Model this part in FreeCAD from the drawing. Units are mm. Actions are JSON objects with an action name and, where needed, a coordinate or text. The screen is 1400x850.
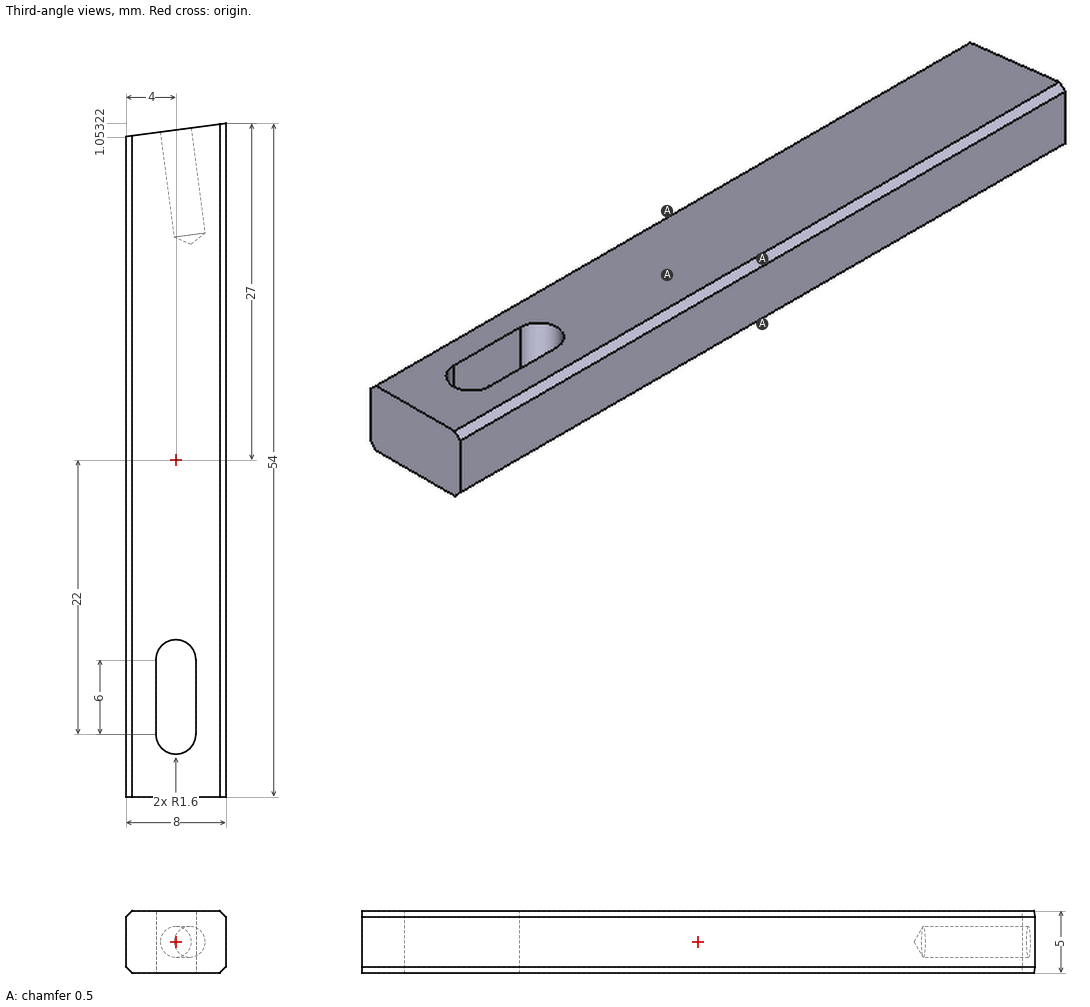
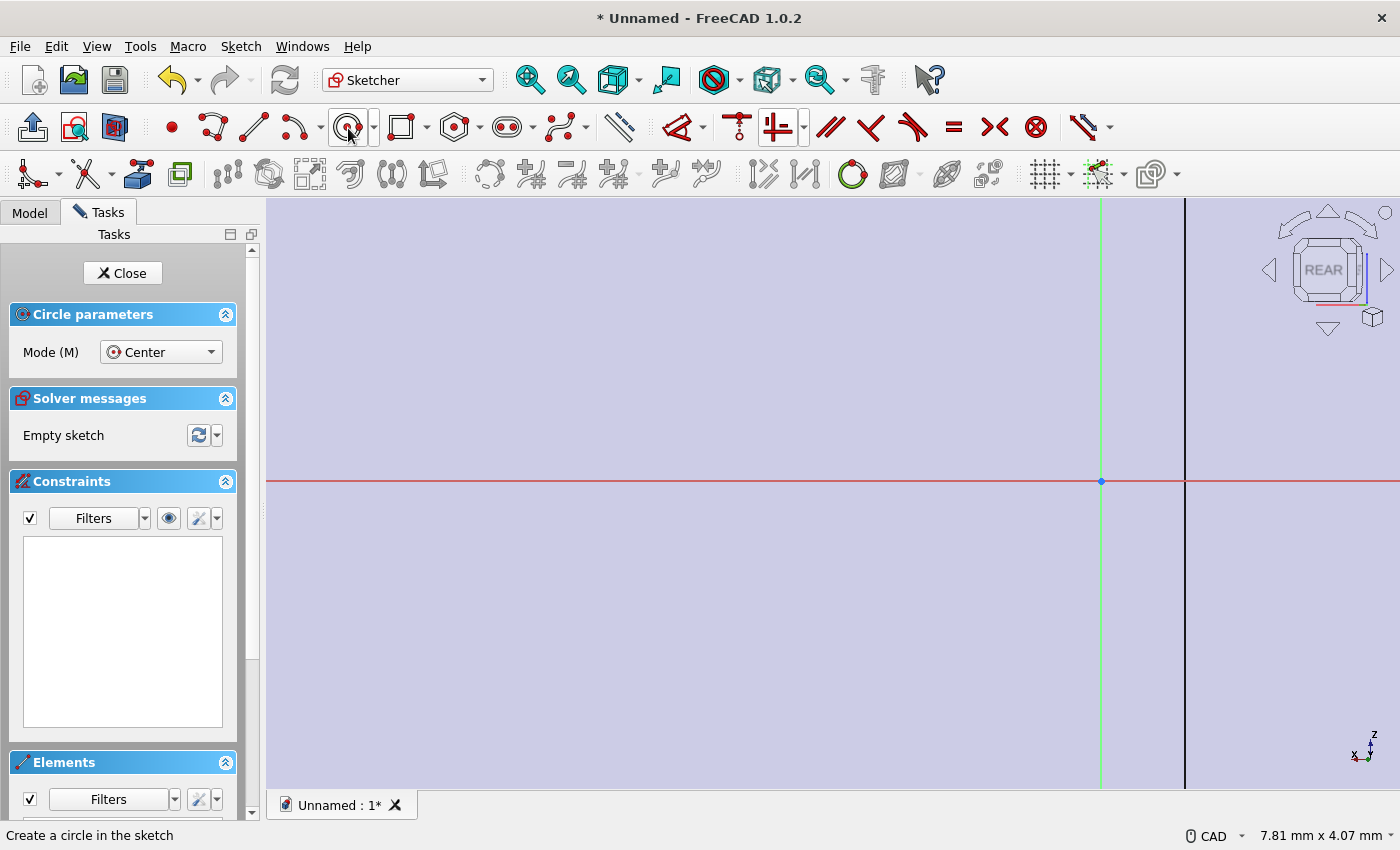
{"action": "left_click", "coordinate": [600, 481]}
{"action": "left_click", "coordinate": [728, 353]}
{"action": "key", "text": "Escape"}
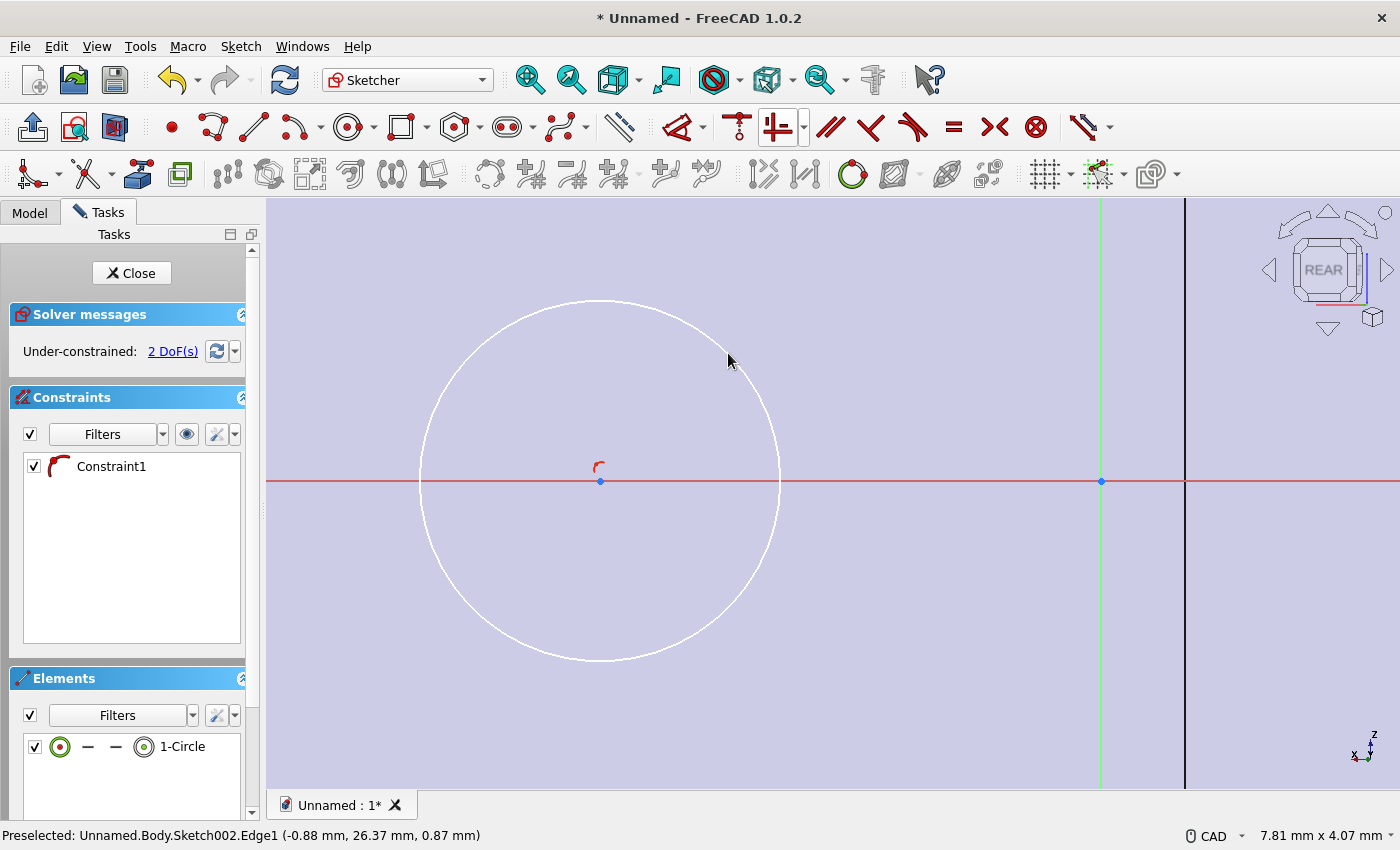
{"action": "left_click", "coordinate": [727, 353]}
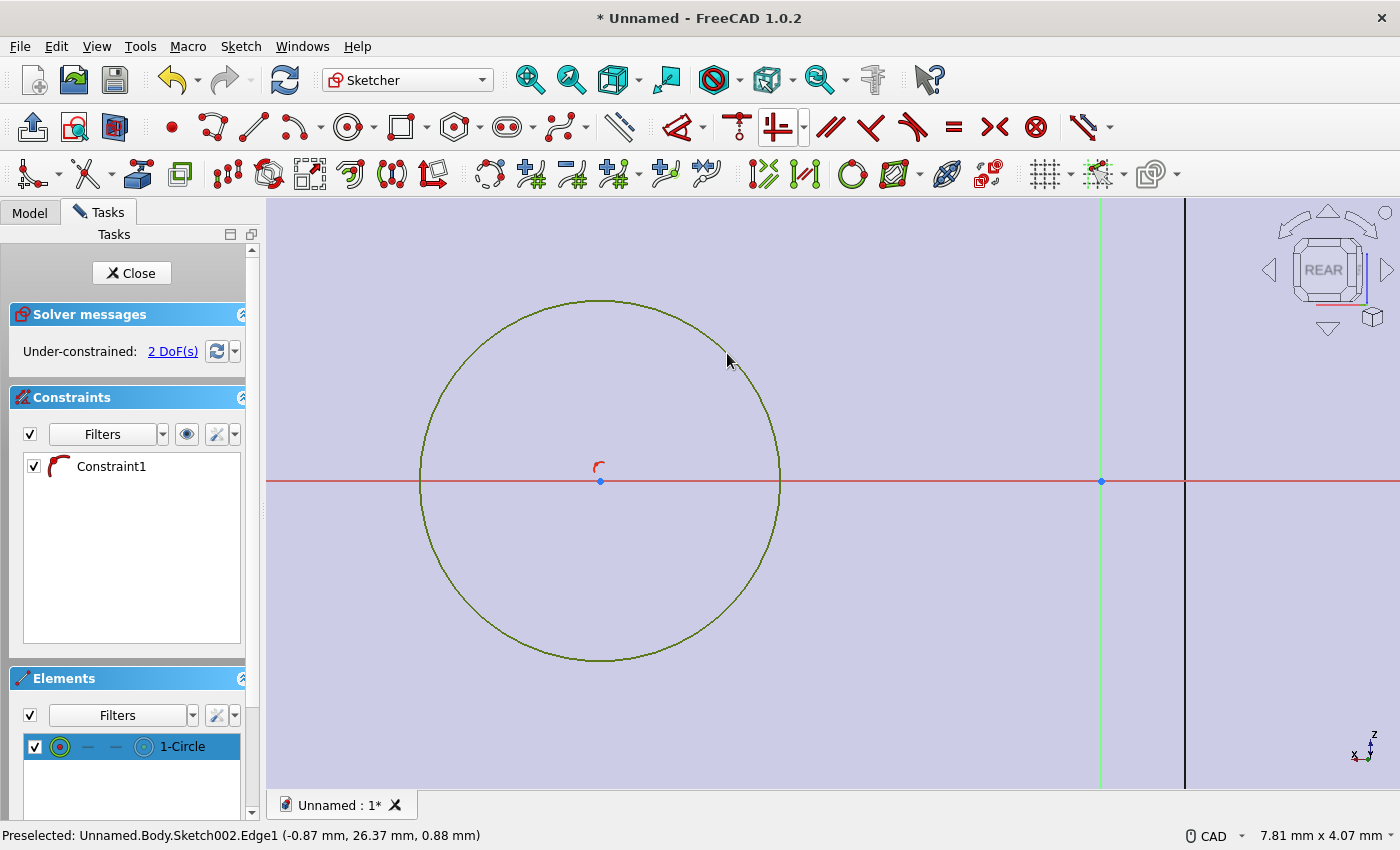
{"action": "left_click", "coordinate": [702, 128]}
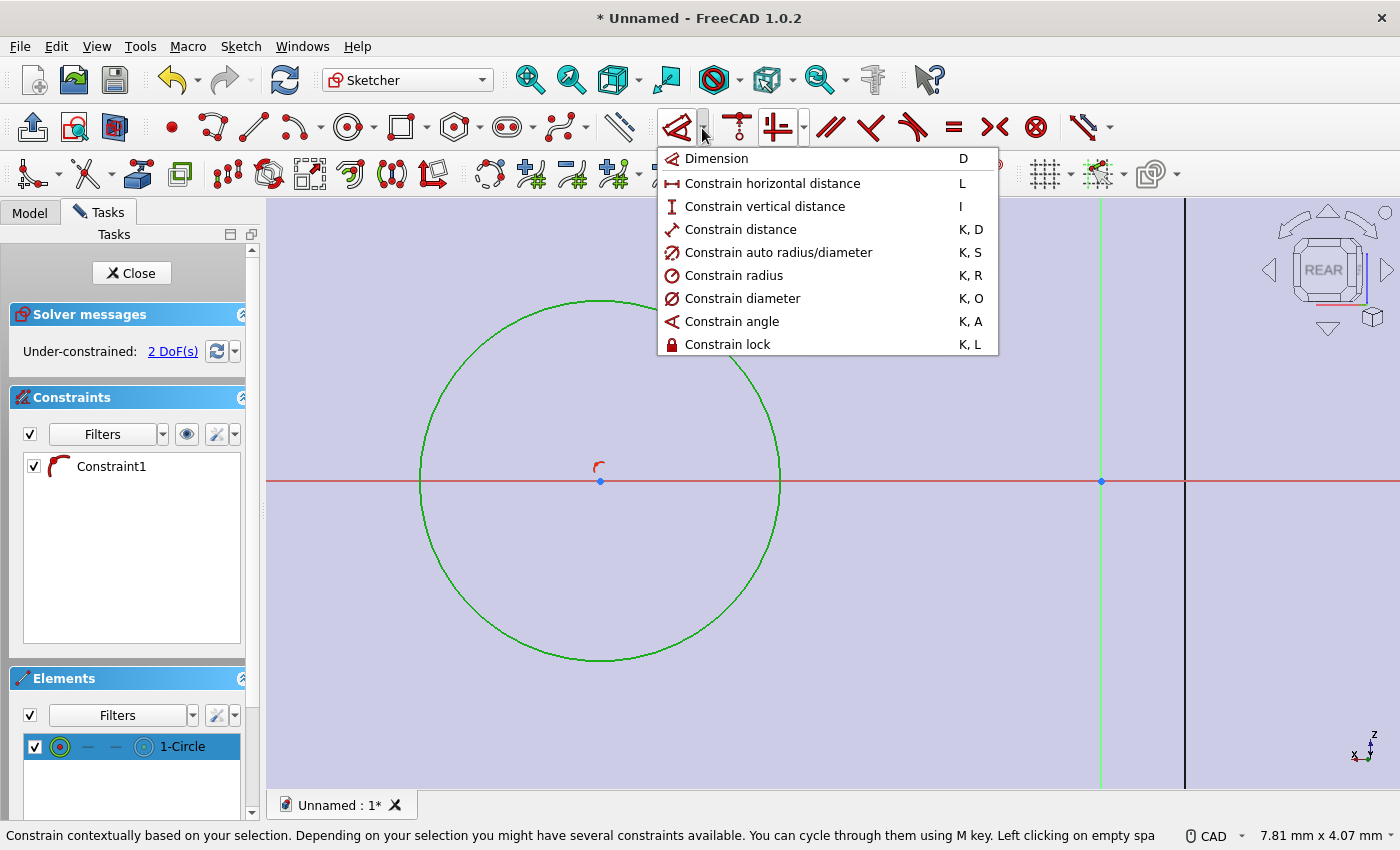
{"action": "left_click", "coordinate": [828, 298]}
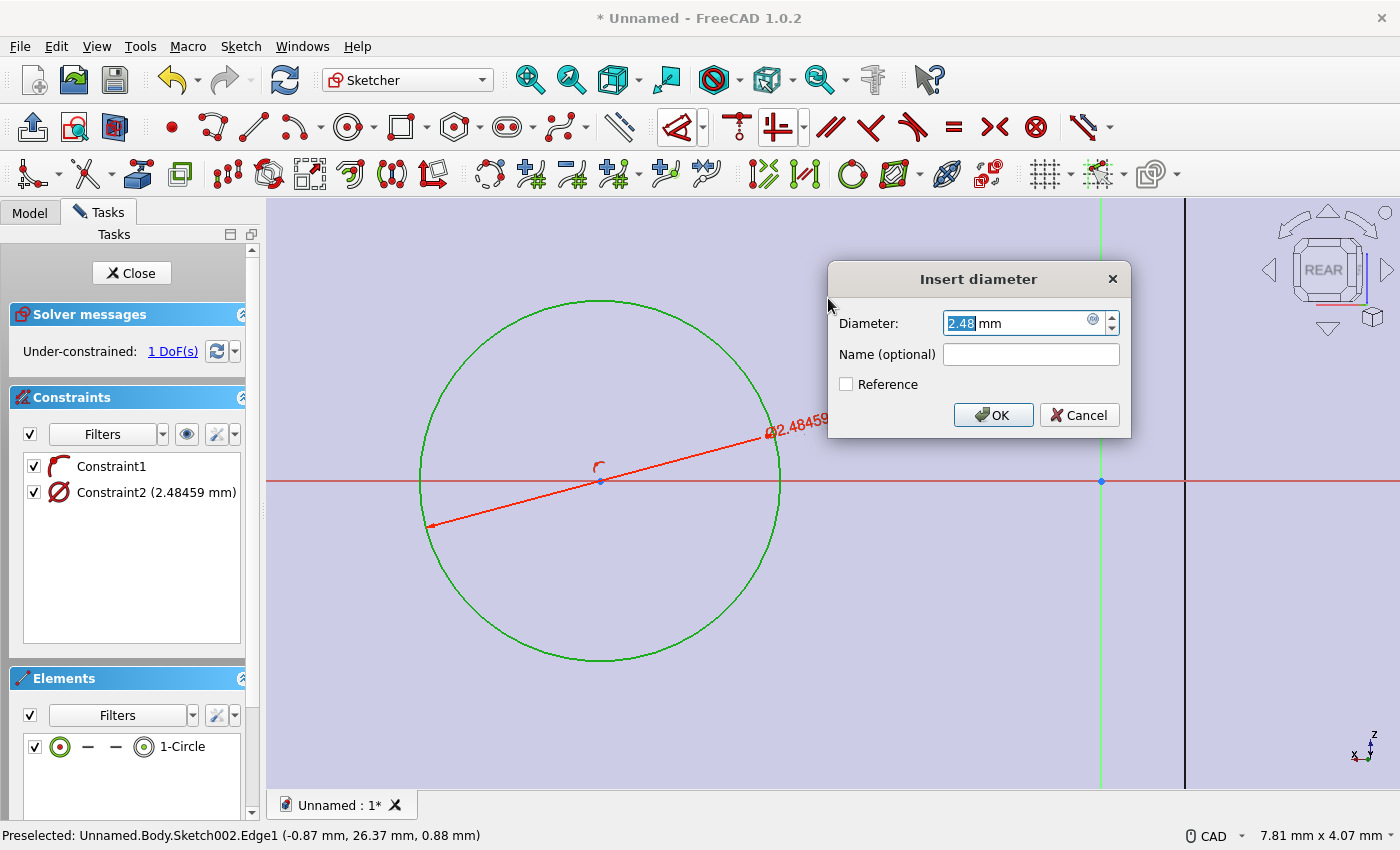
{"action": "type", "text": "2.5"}
{"action": "key", "text": "Return"}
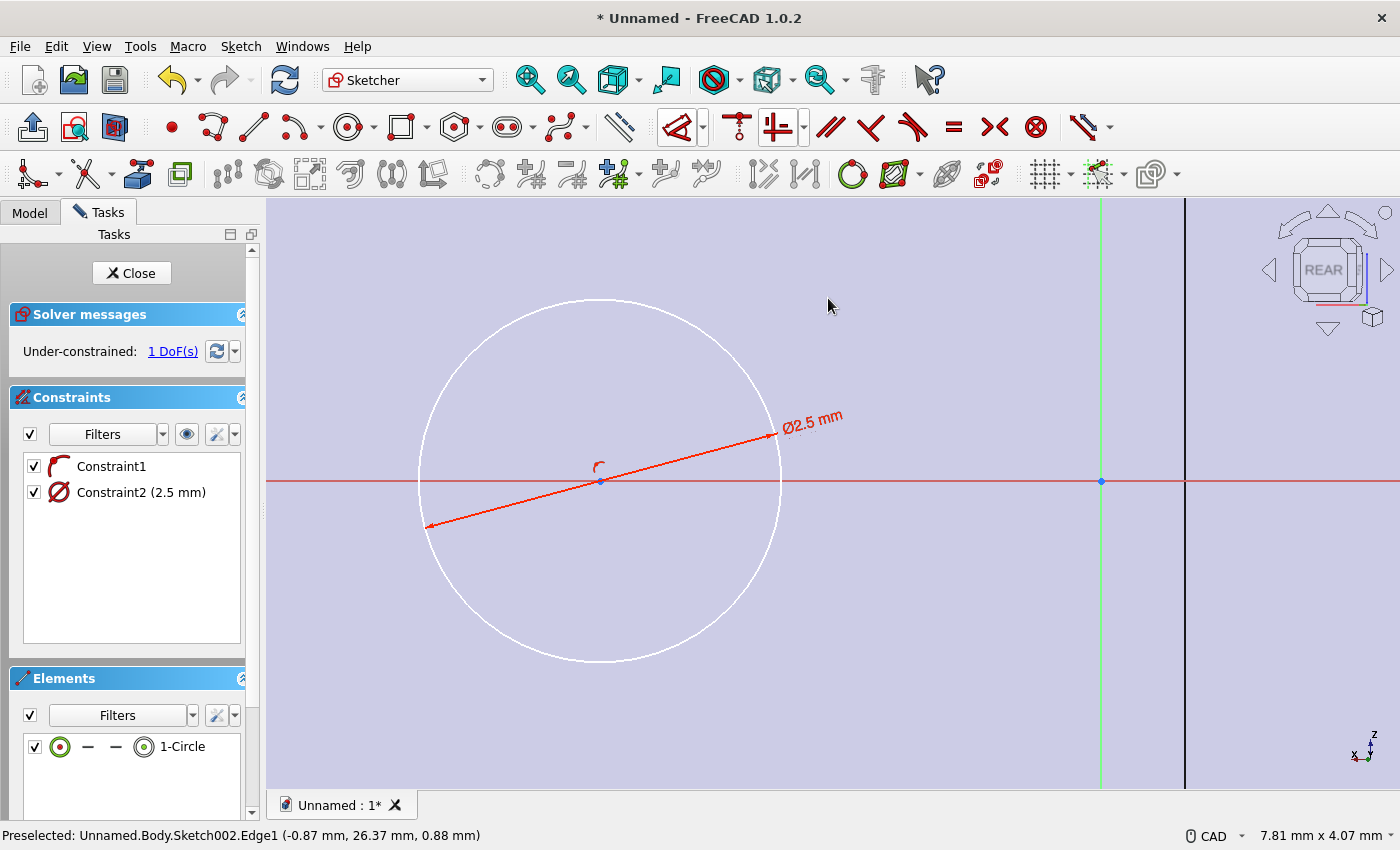
{"action": "left_click", "coordinate": [600, 481]}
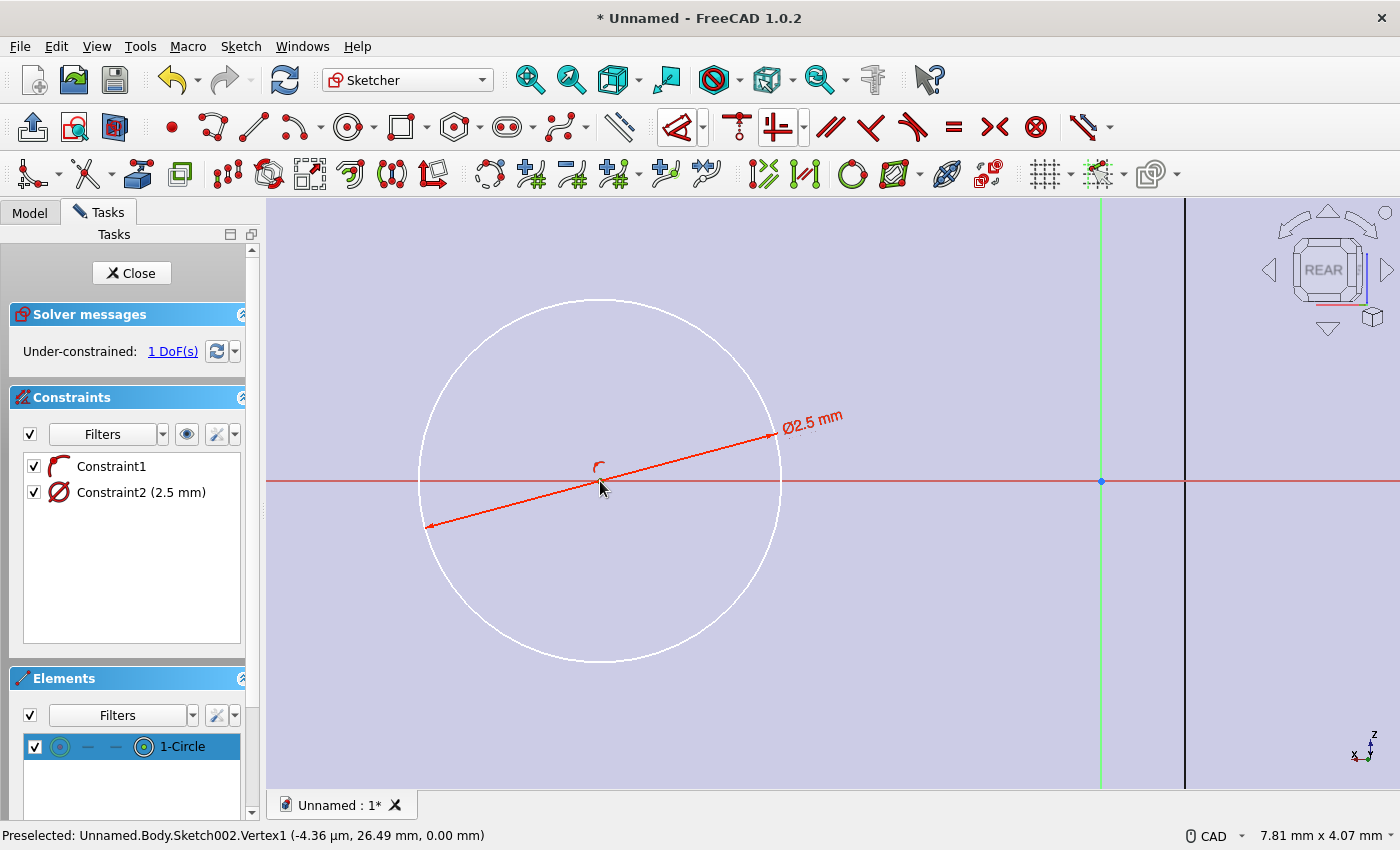
{"action": "key", "text": "l"}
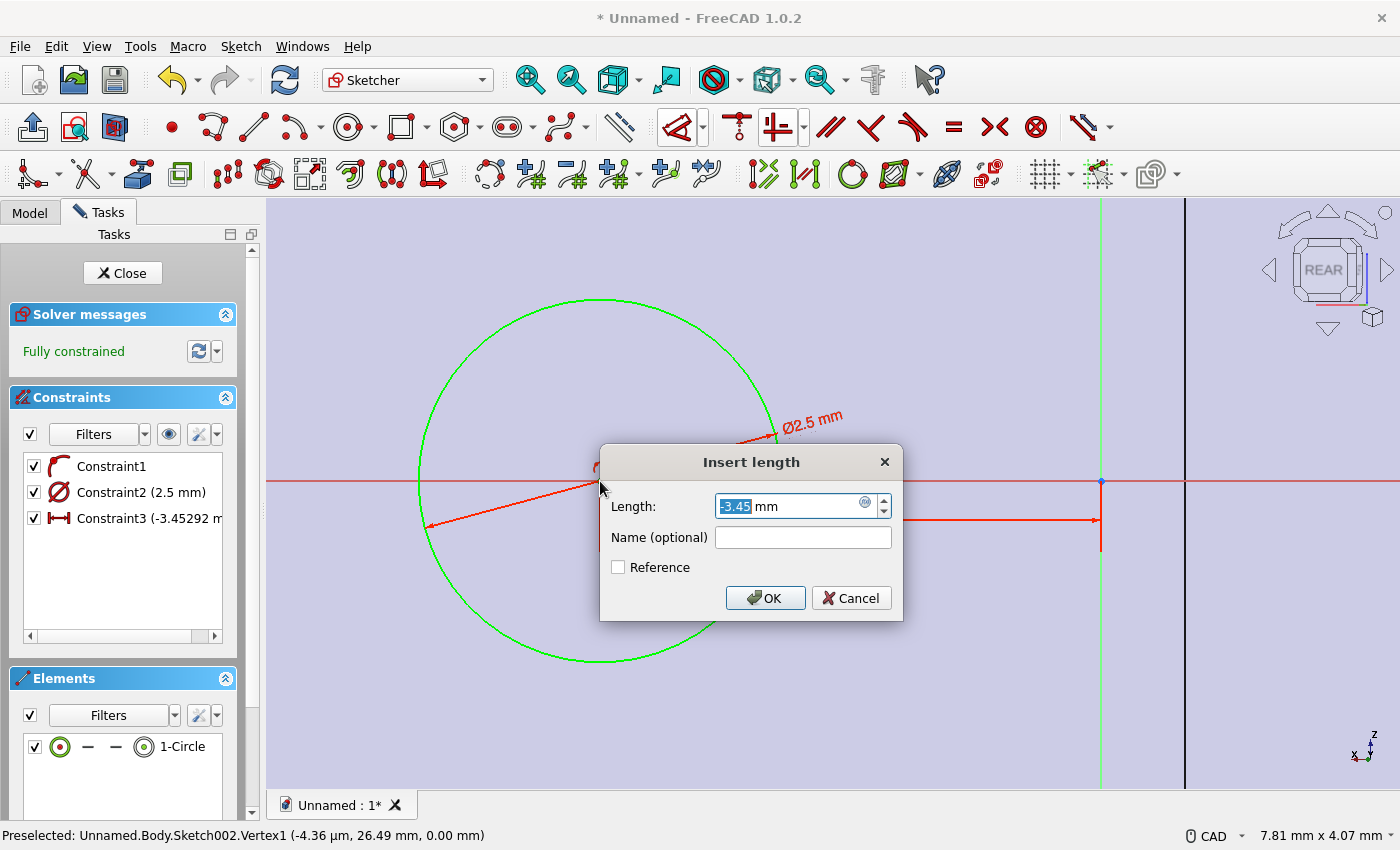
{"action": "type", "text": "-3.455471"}
{"action": "key", "text": "Return"}